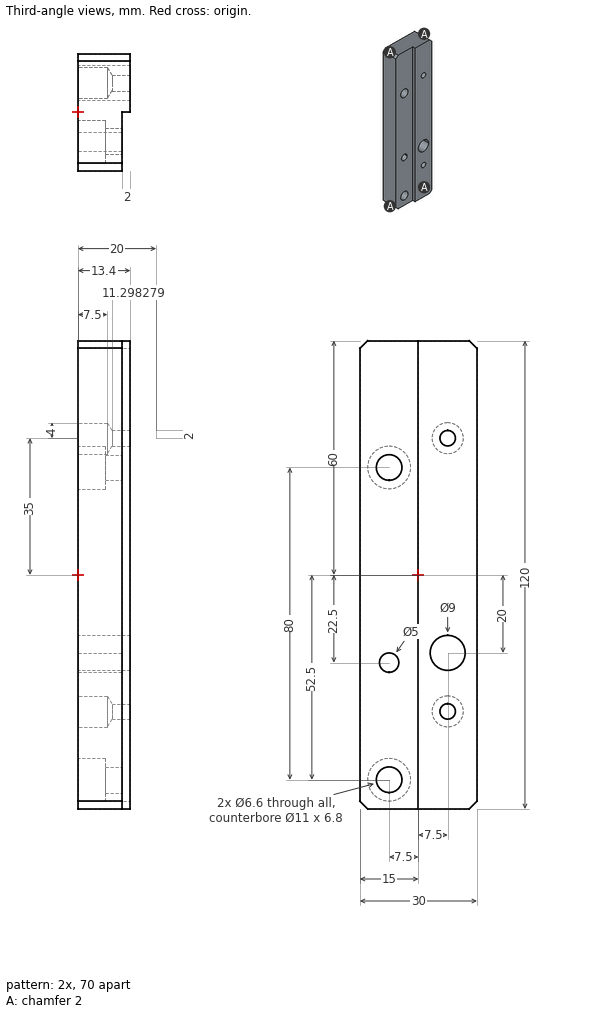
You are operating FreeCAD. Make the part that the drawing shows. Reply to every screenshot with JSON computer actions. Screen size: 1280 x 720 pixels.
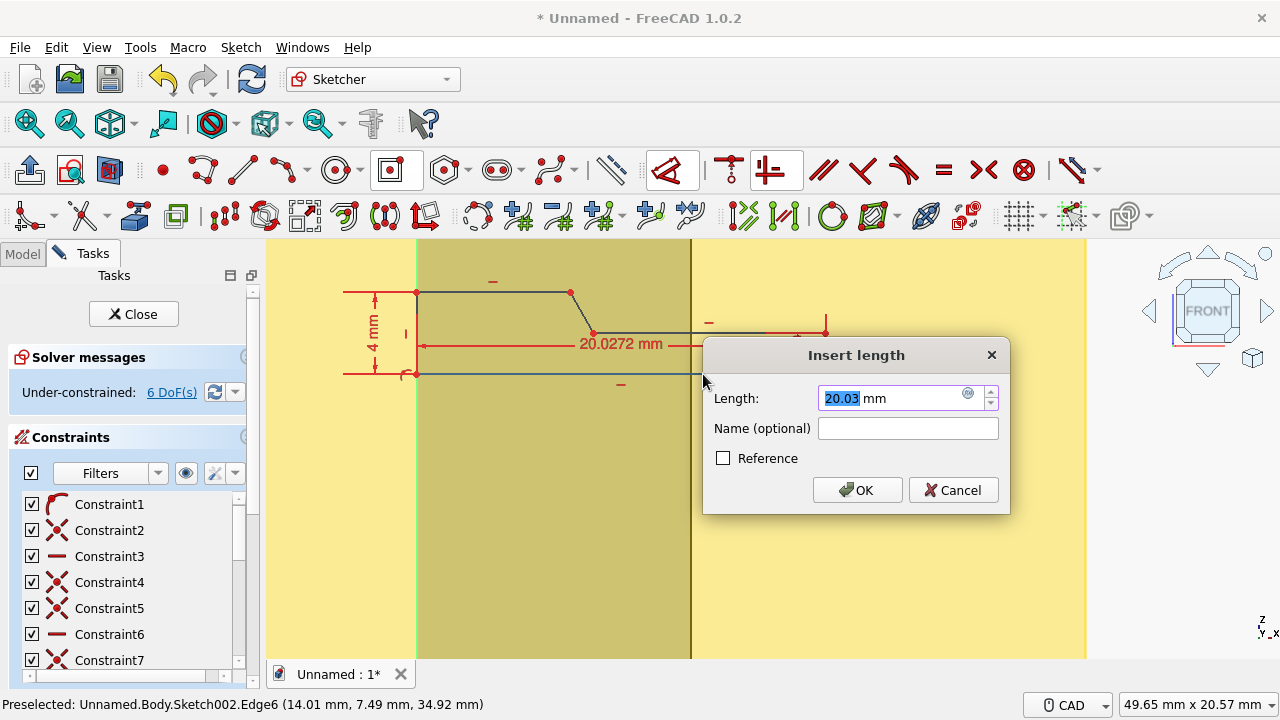
{"action": "type", "text": "20"}
{"action": "key", "text": "Return"}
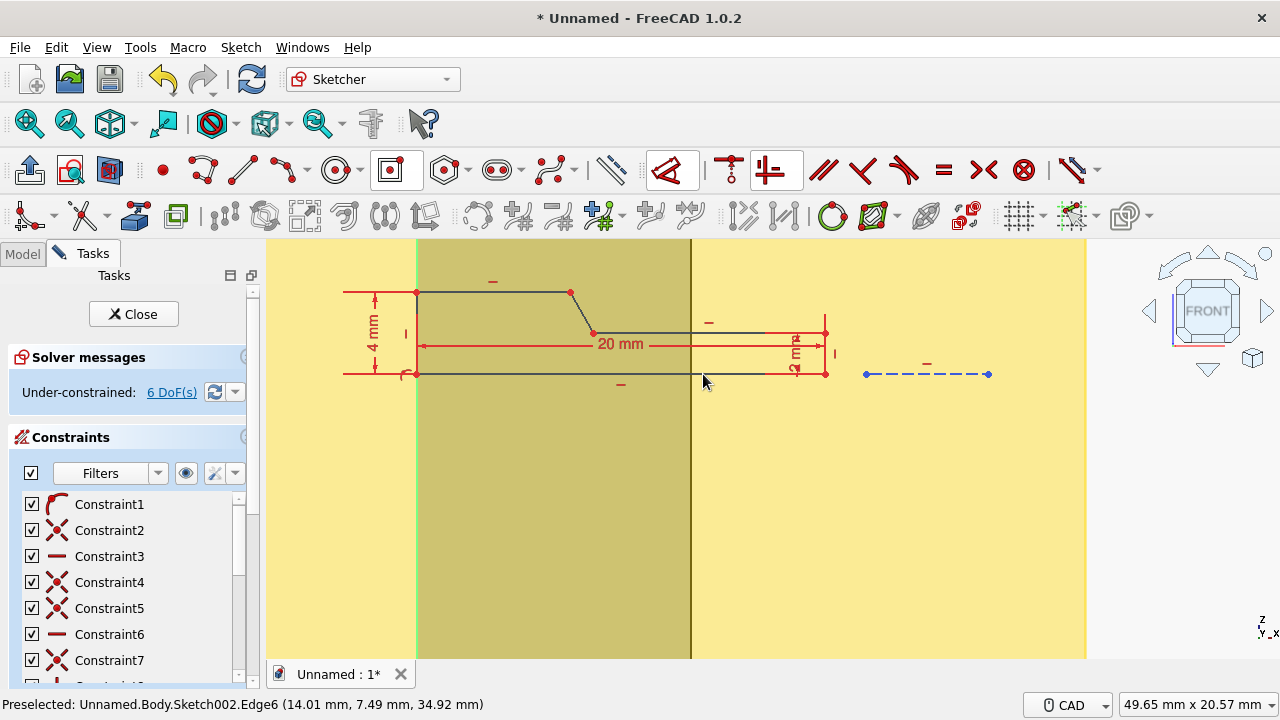
{"action": "left_click", "coordinate": [463, 292]}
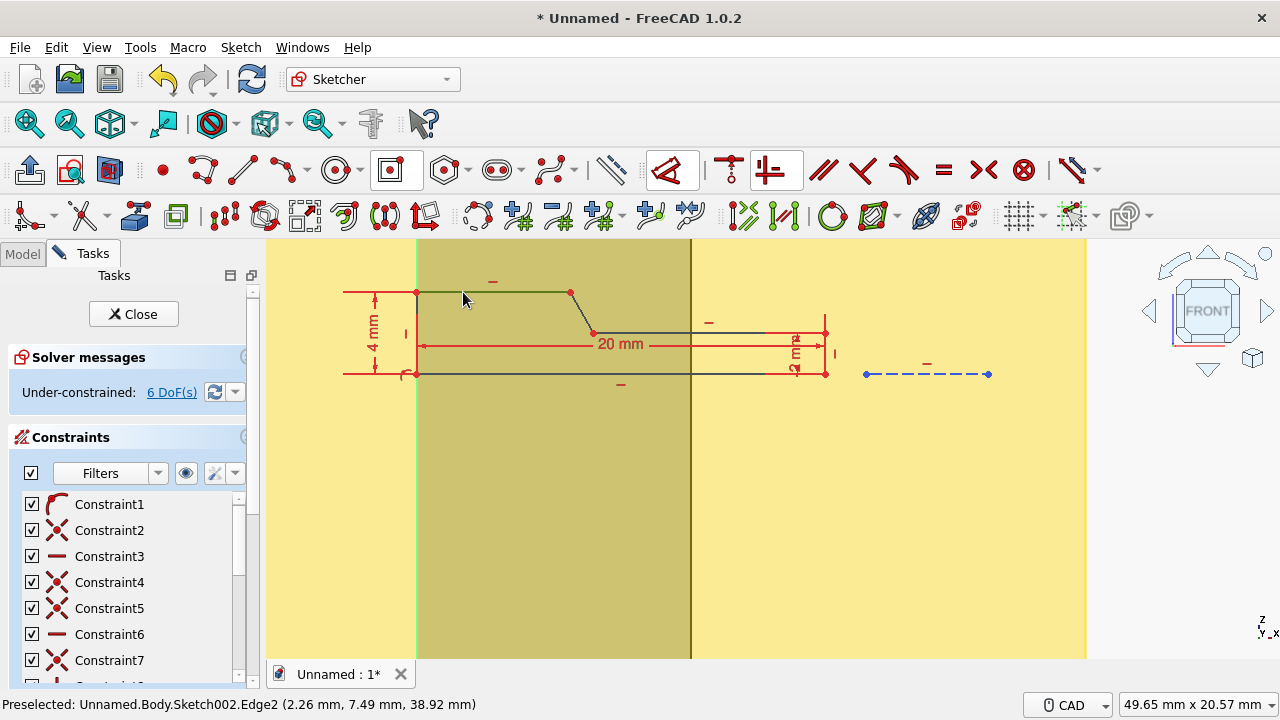
{"action": "key", "text": "l"}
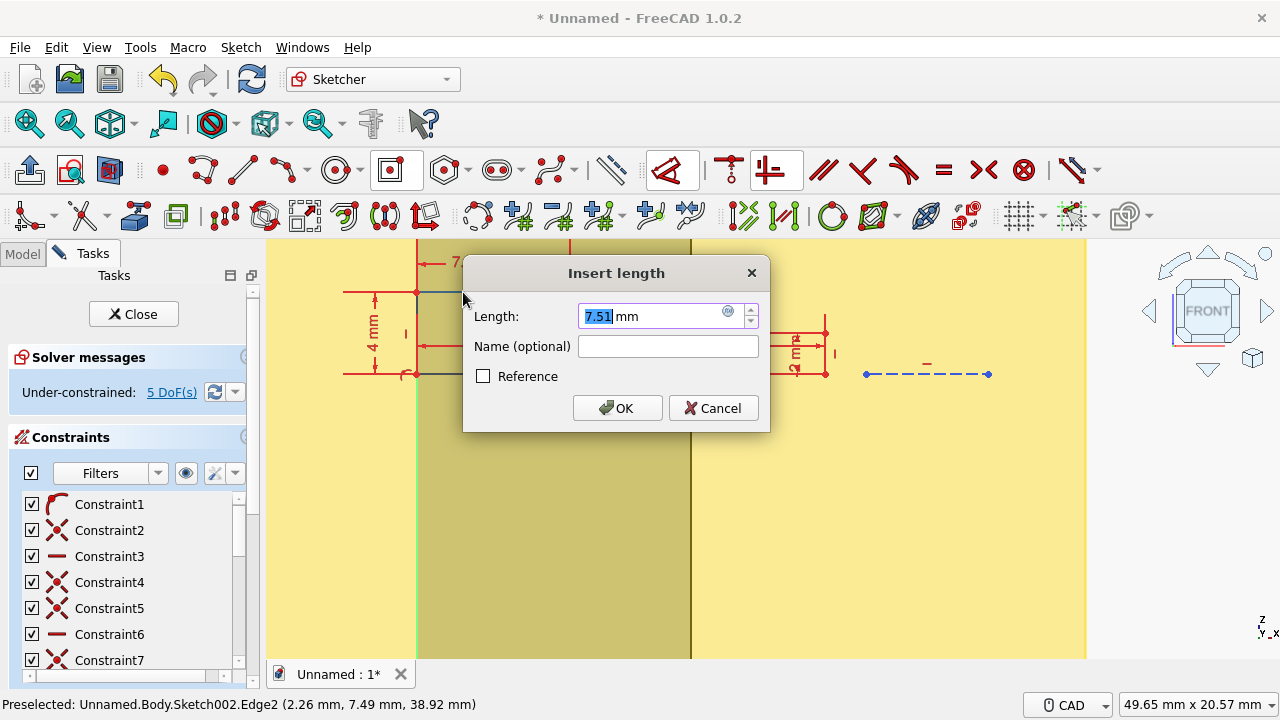
{"action": "type", "text": "7.5"}
{"action": "key", "text": "Return"}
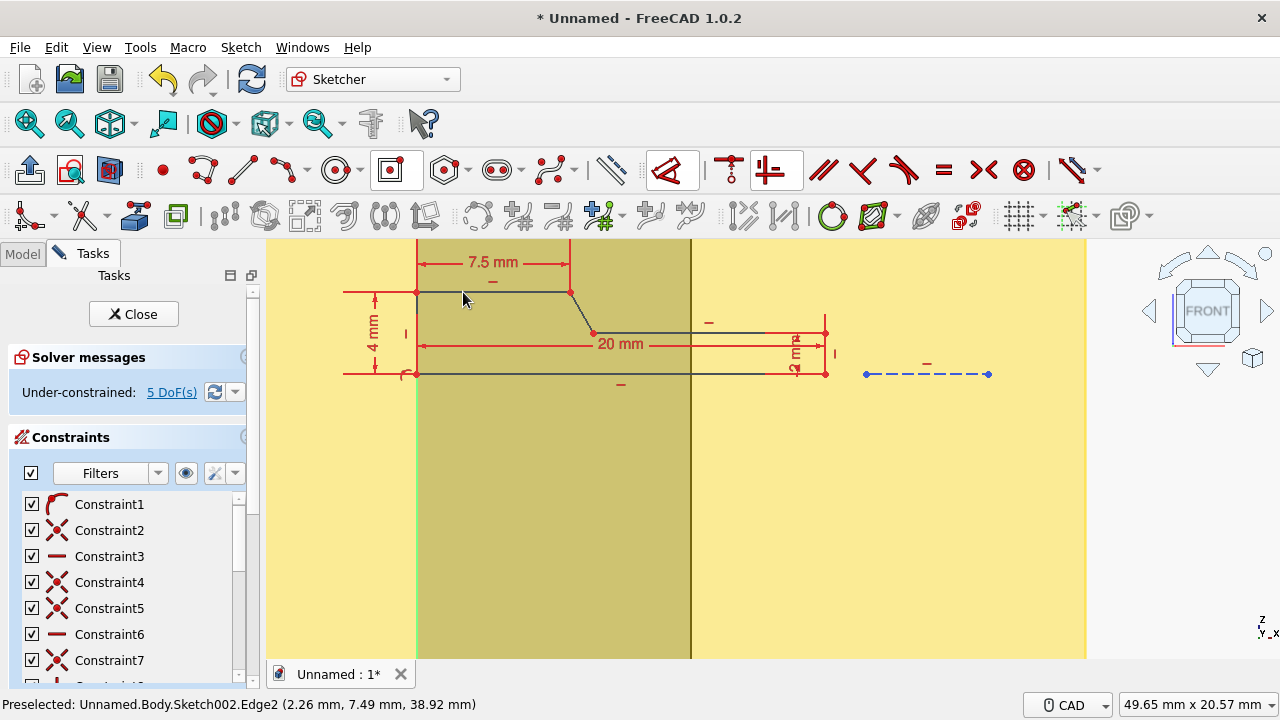
{"action": "left_click", "coordinate": [417, 374]}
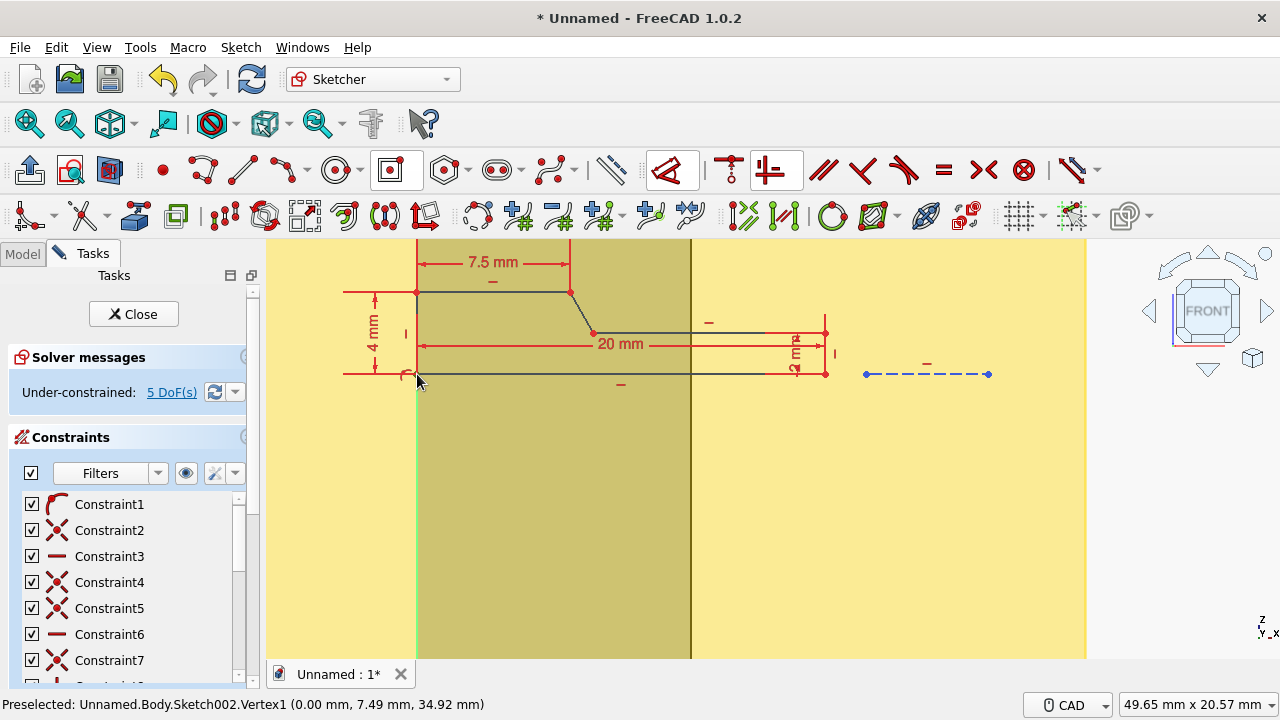
{"action": "key", "text": "i"}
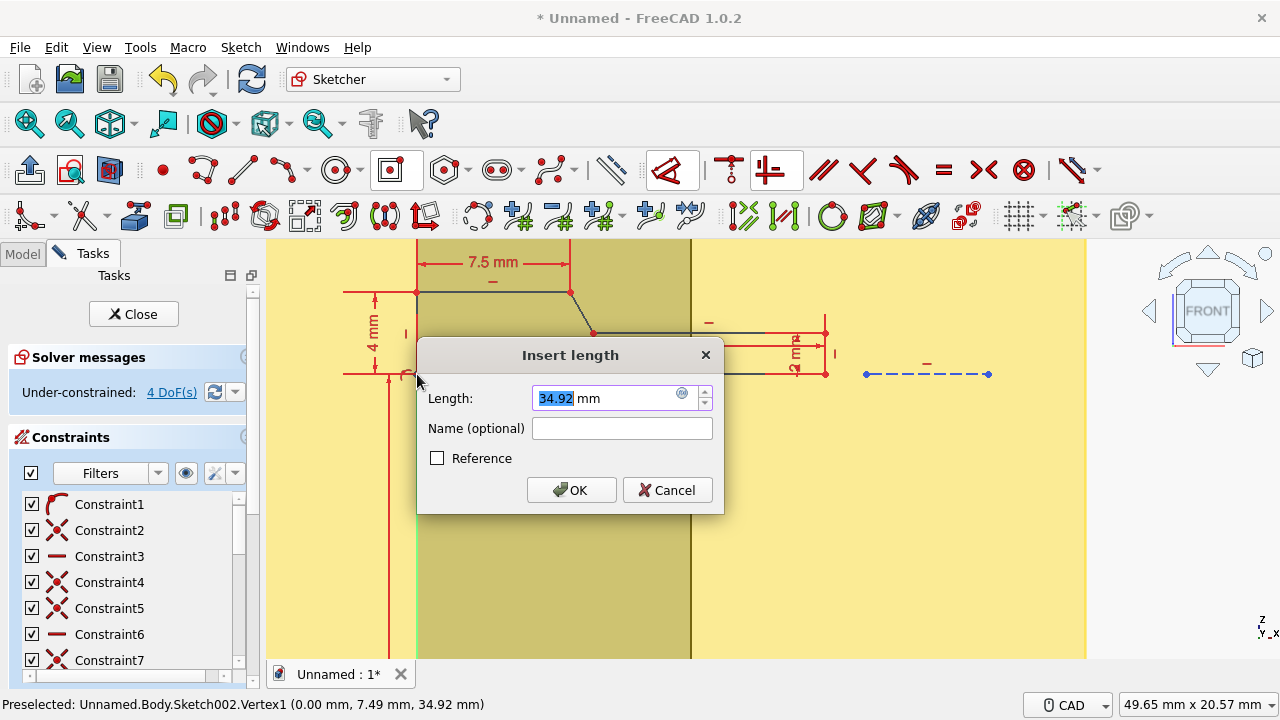
{"action": "type", "text": "35"}
{"action": "key", "text": "Return"}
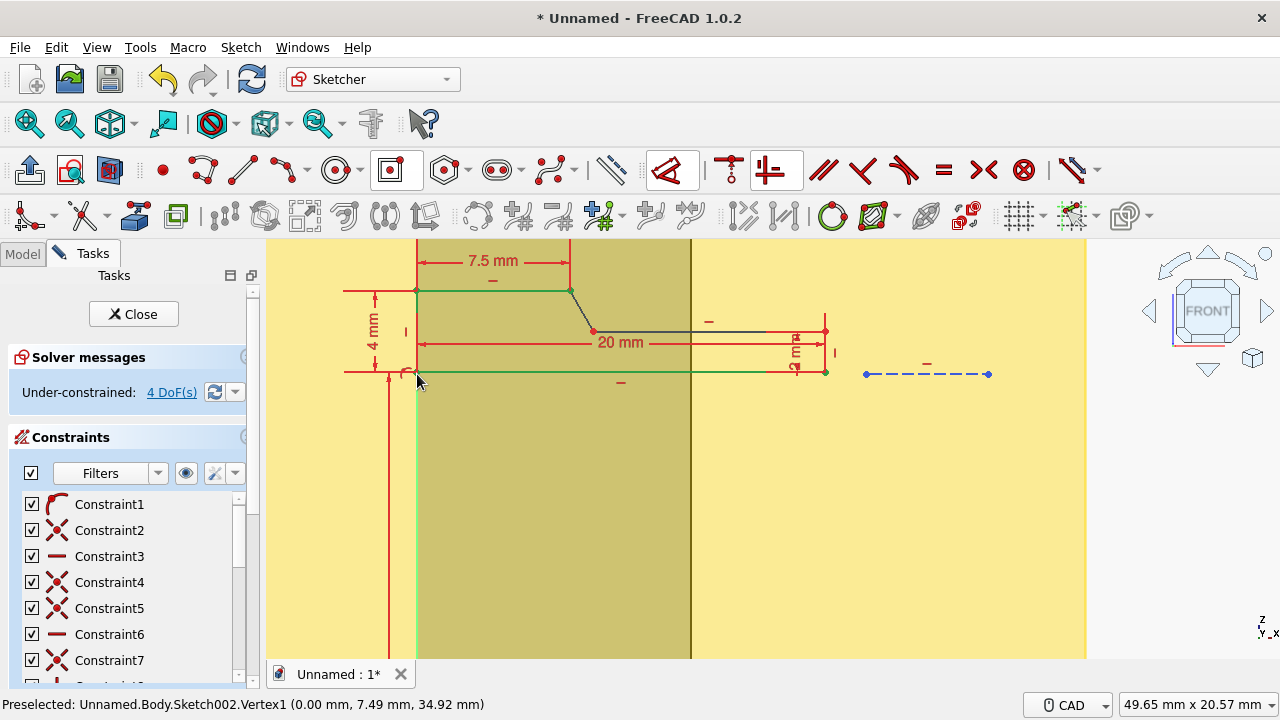
{"action": "left_click", "coordinate": [866, 374]}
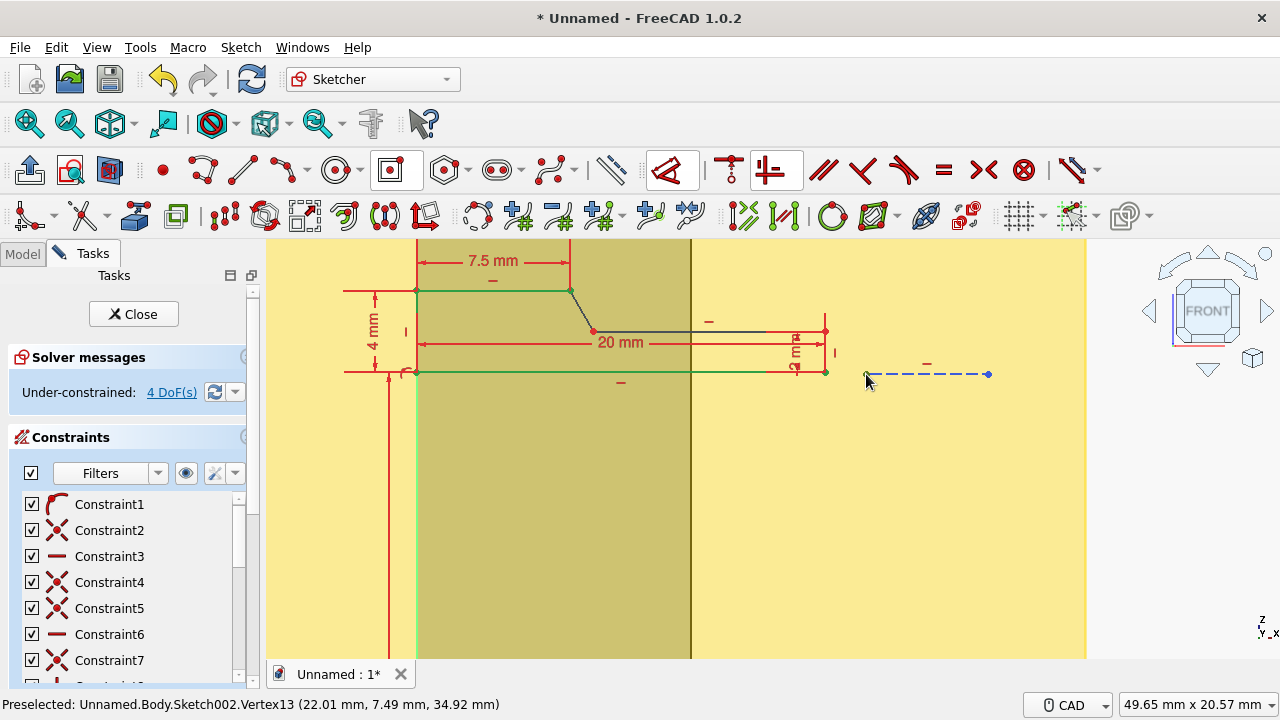
{"action": "left_click", "coordinate": [694, 170]}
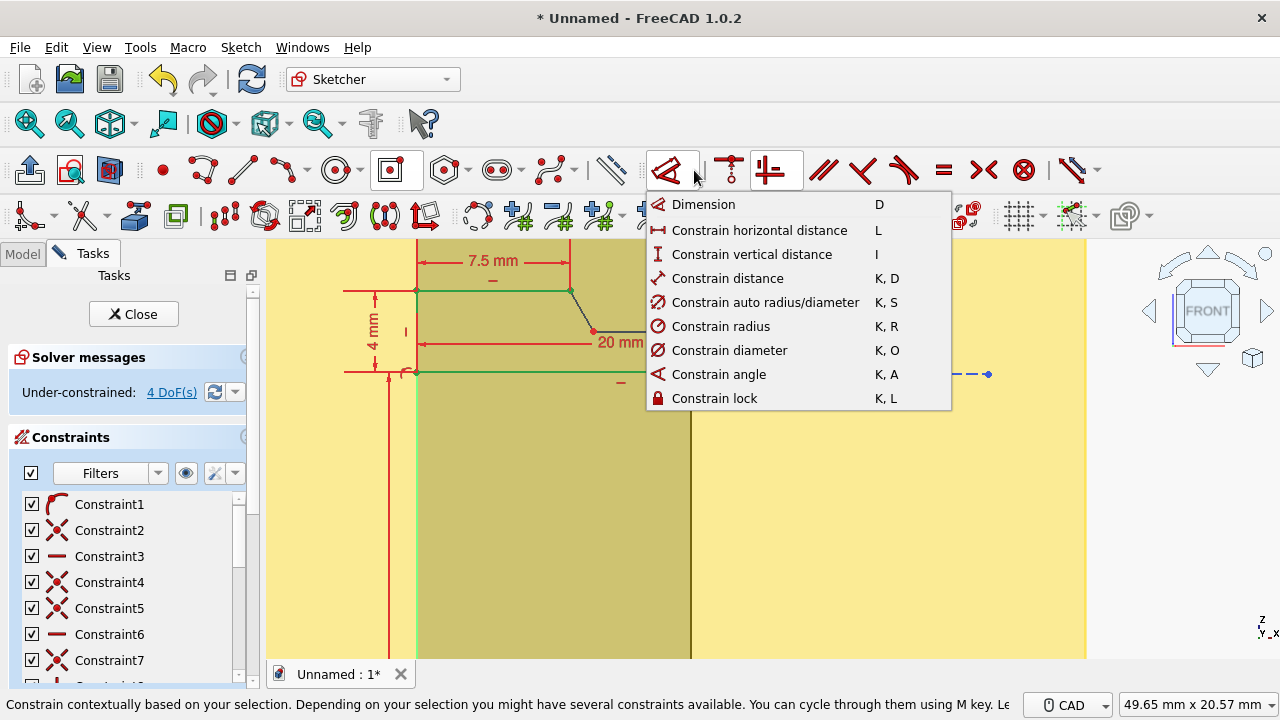
{"action": "left_click", "coordinate": [799, 254]}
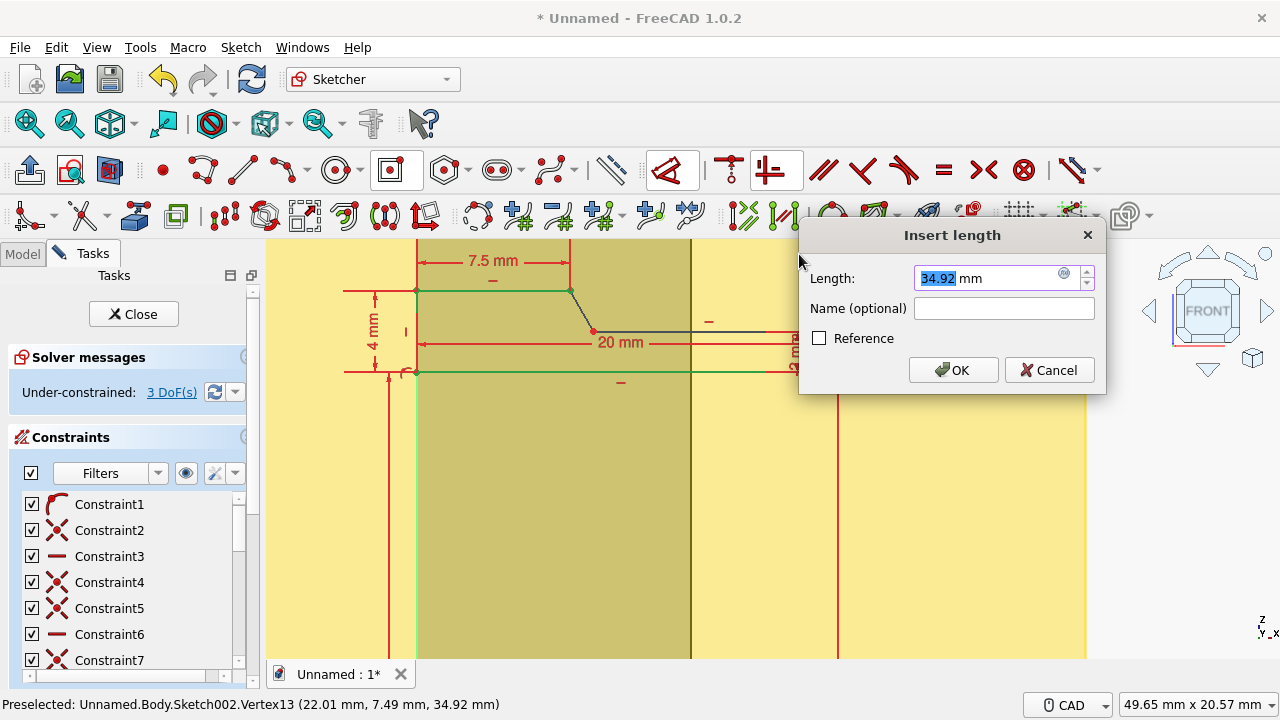
{"action": "type", "text": "35"}
{"action": "key", "text": "Return"}